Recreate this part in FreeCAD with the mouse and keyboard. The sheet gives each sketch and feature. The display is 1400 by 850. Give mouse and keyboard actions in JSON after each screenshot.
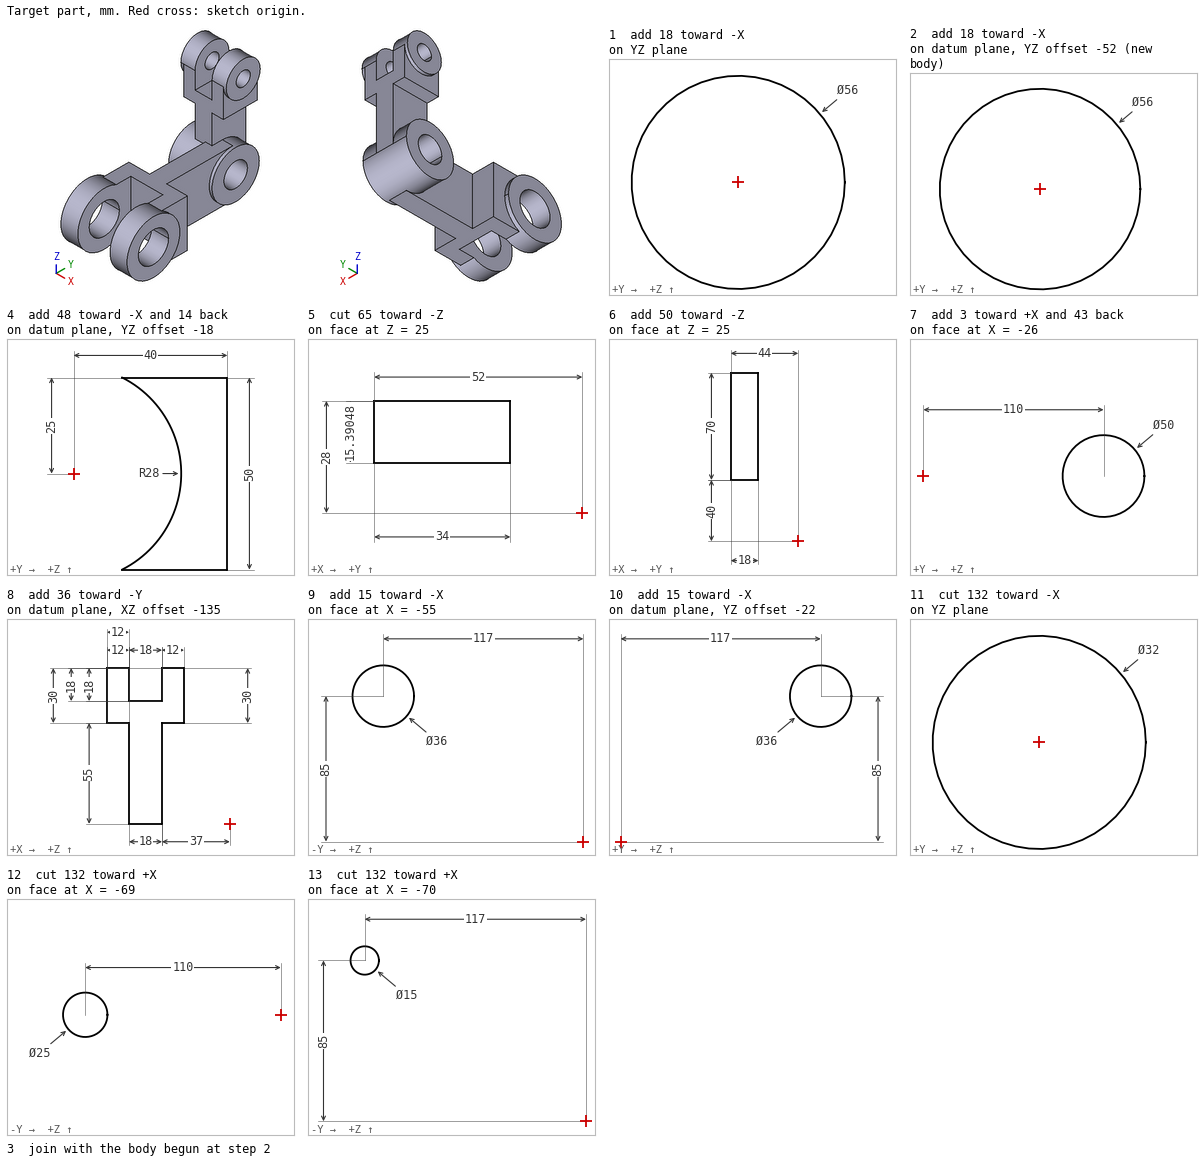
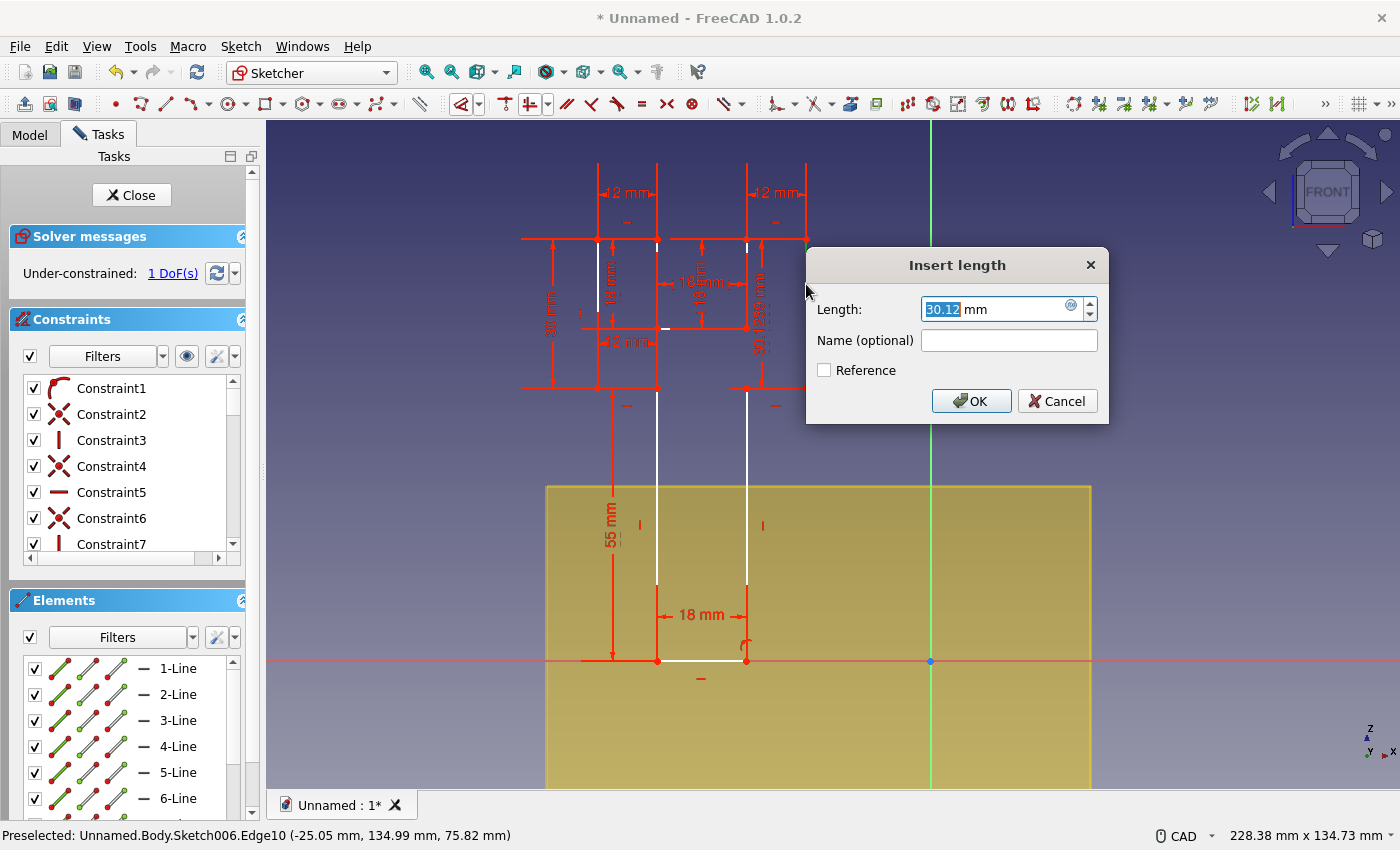
{"action": "type", "text": "30"}
{"action": "key", "text": "Return"}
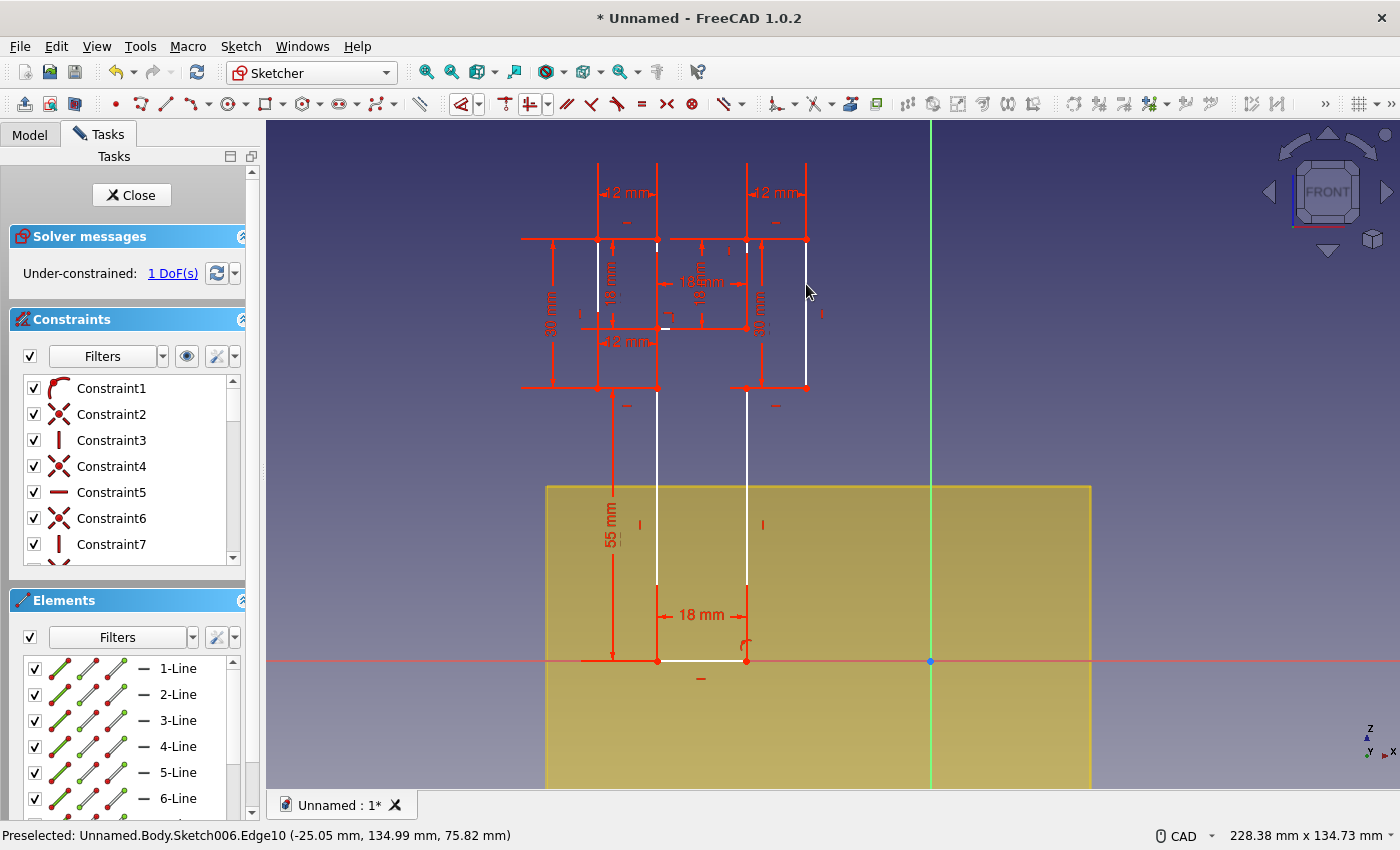
{"action": "left_click", "coordinate": [747, 661]}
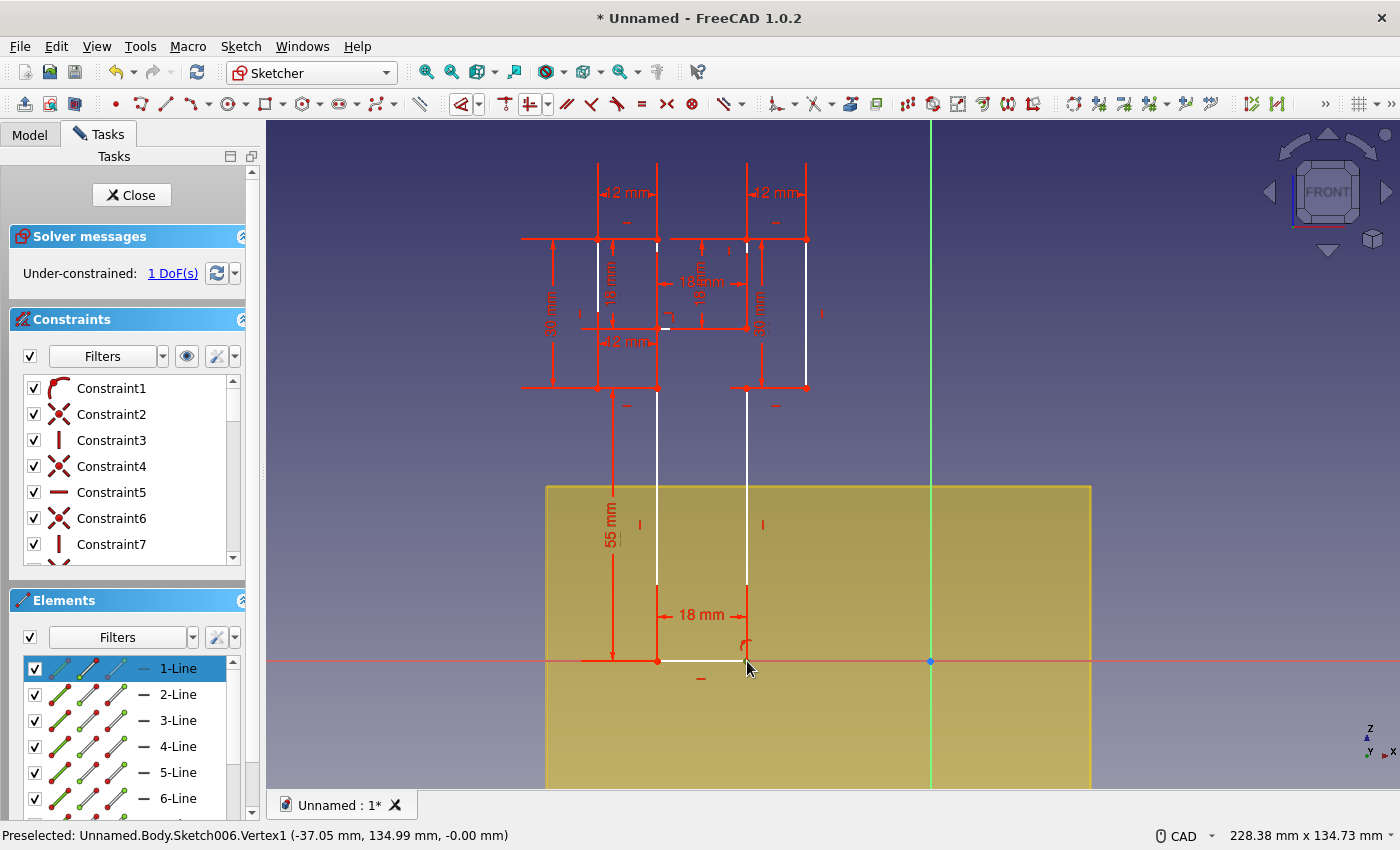
{"action": "left_click", "coordinate": [478, 104]}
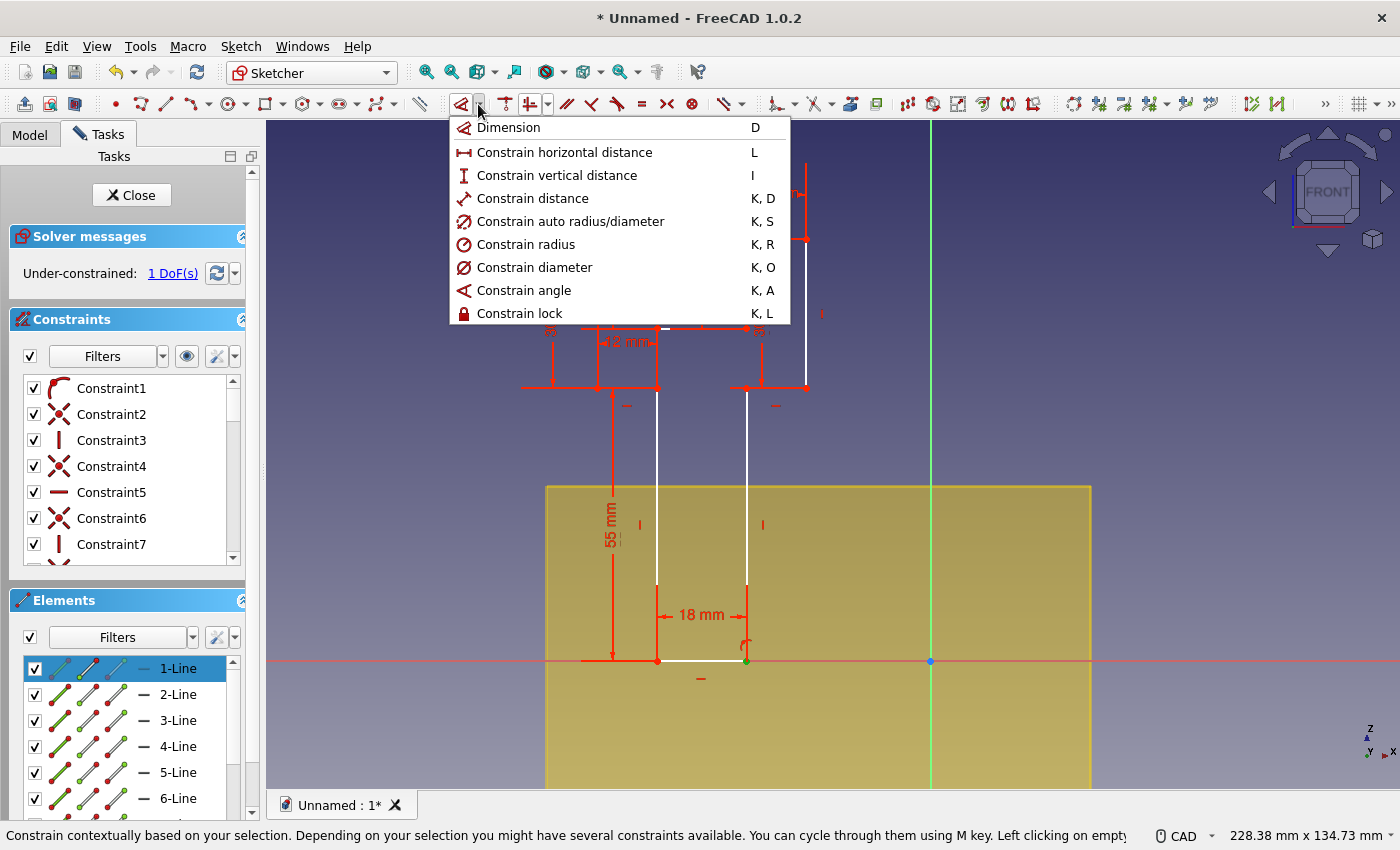
{"action": "left_click", "coordinate": [620, 152]}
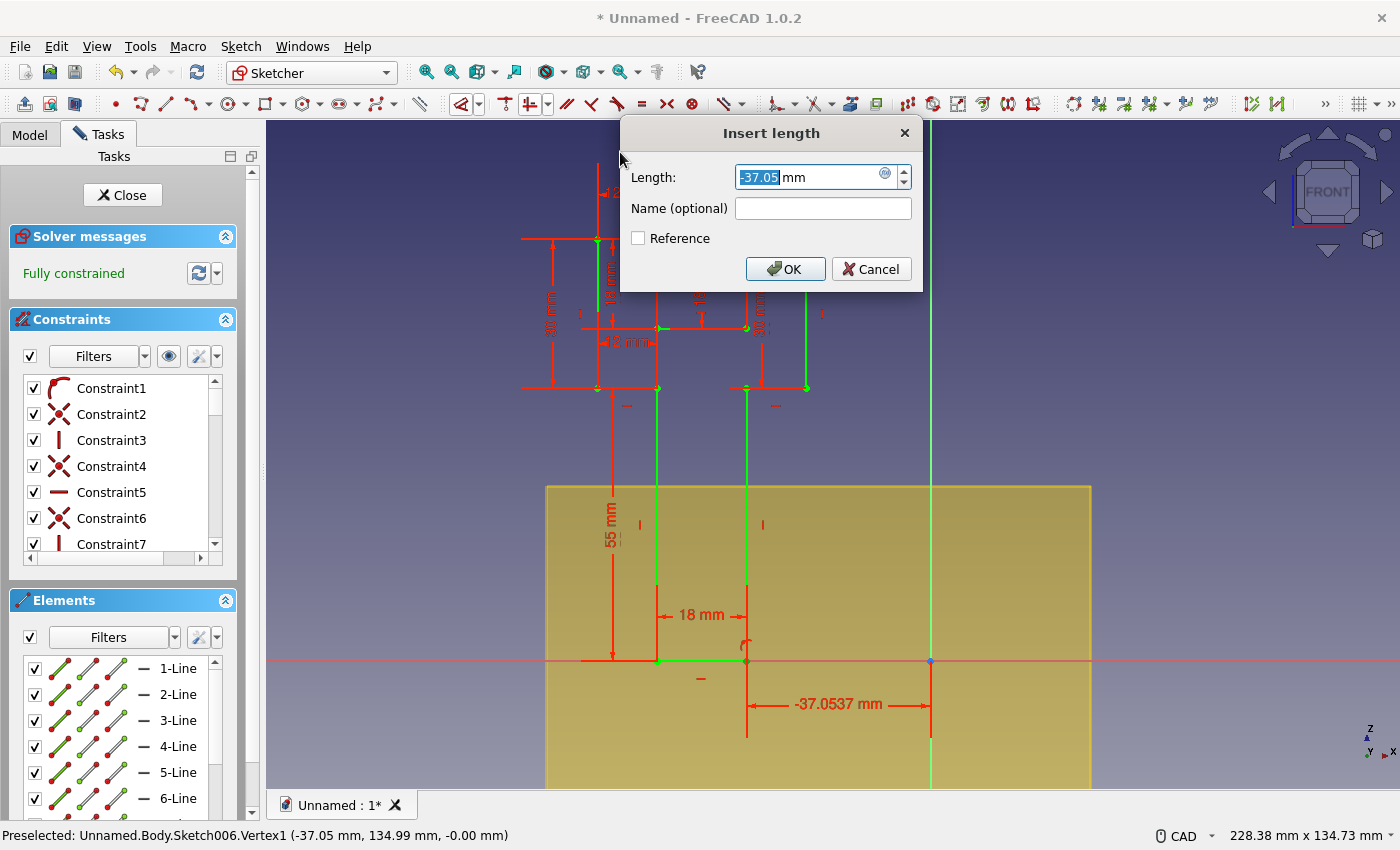
{"action": "type", "text": "-37"}
{"action": "key", "text": "Return"}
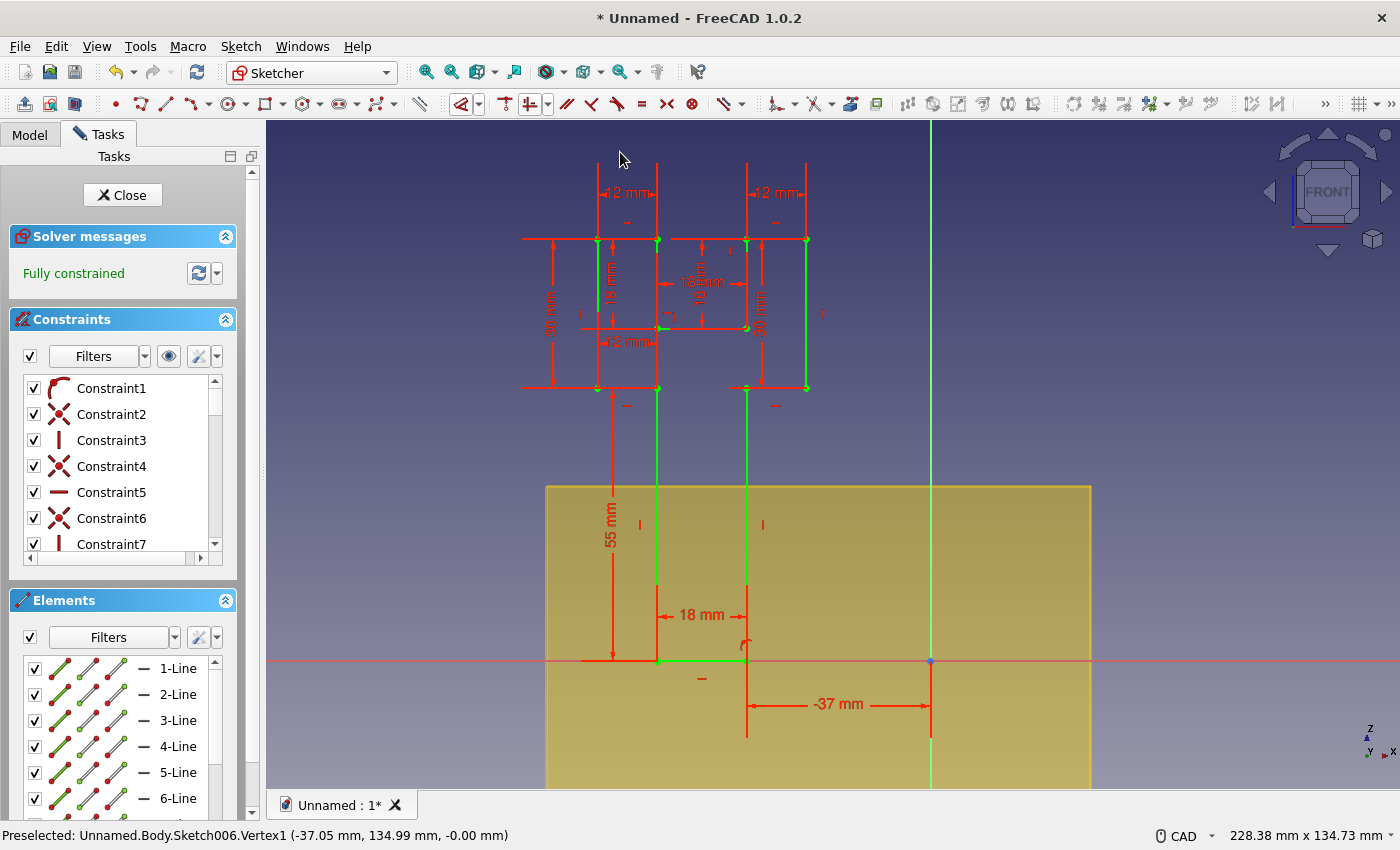
{"action": "left_click", "coordinate": [123, 195]}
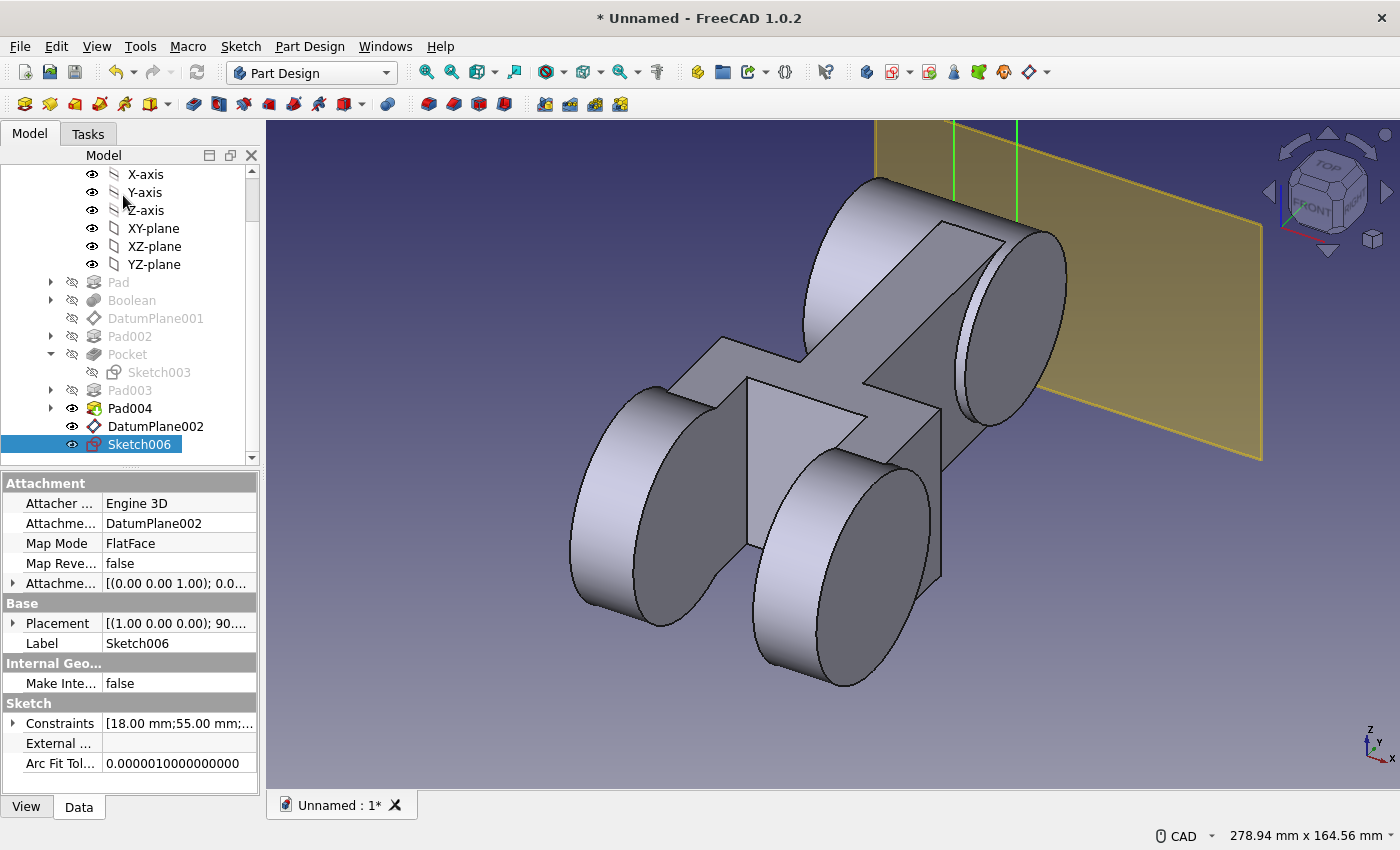
{"action": "left_click", "coordinate": [25, 104]}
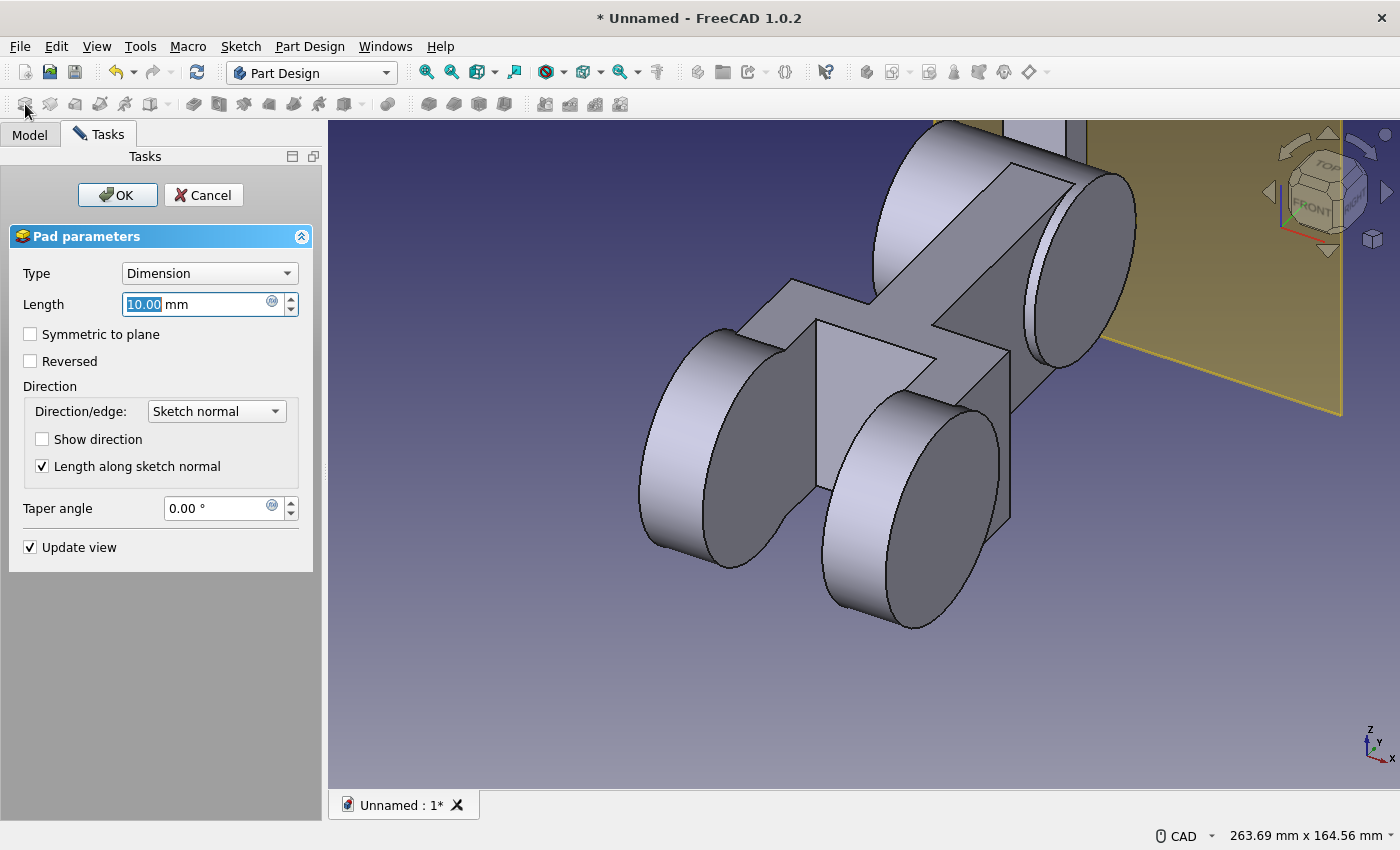
{"action": "type", "text": "36"}
{"action": "key", "text": "Tab"}